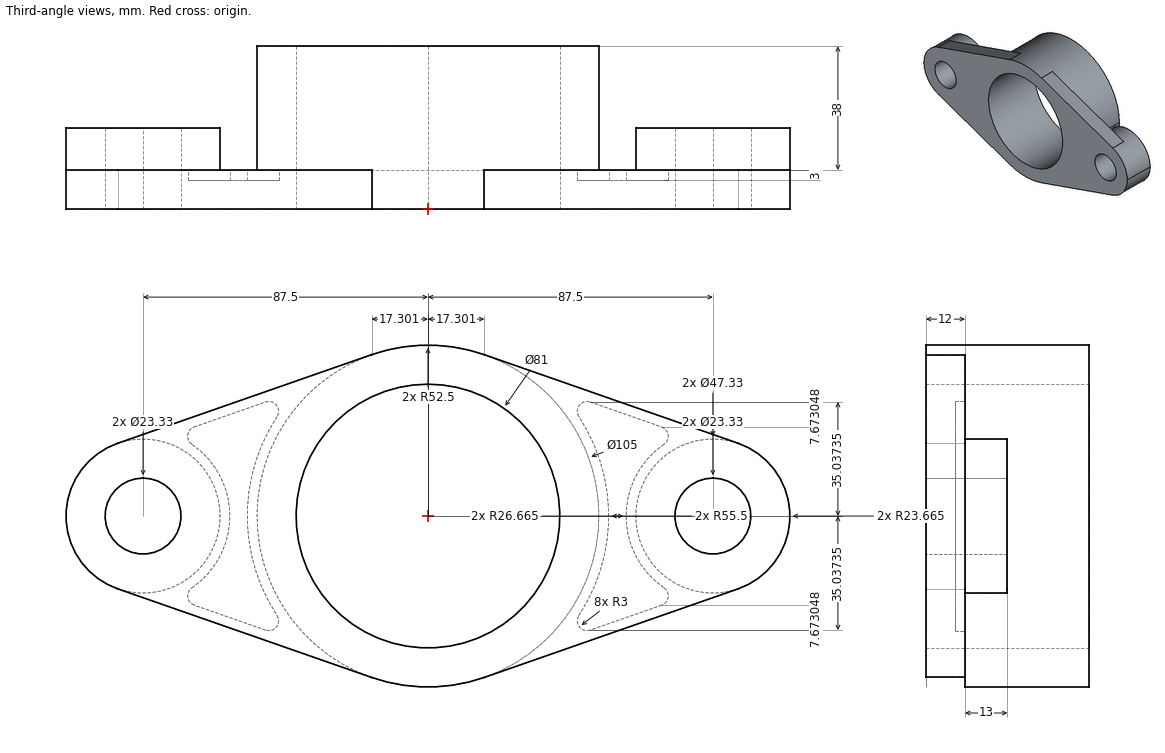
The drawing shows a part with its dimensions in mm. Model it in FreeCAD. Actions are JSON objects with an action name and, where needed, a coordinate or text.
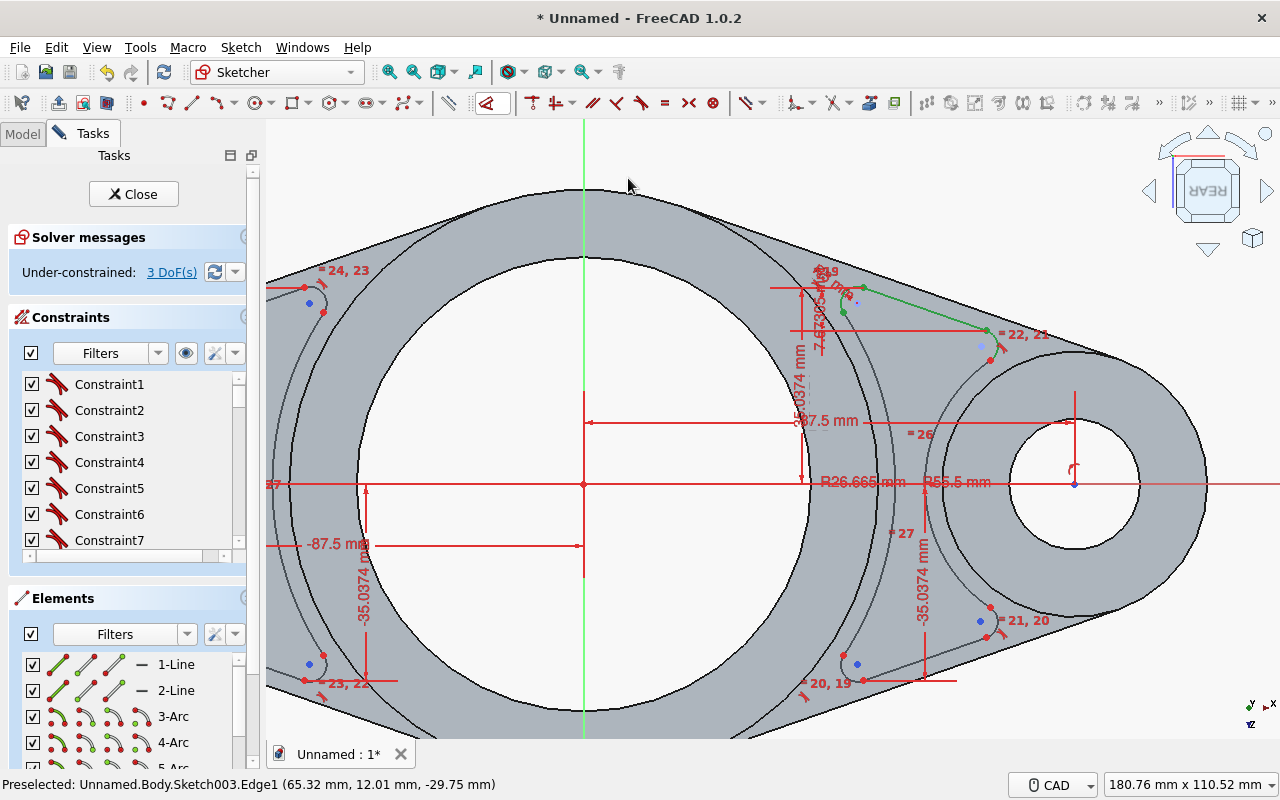
{"action": "left_click", "coordinate": [900, 668]}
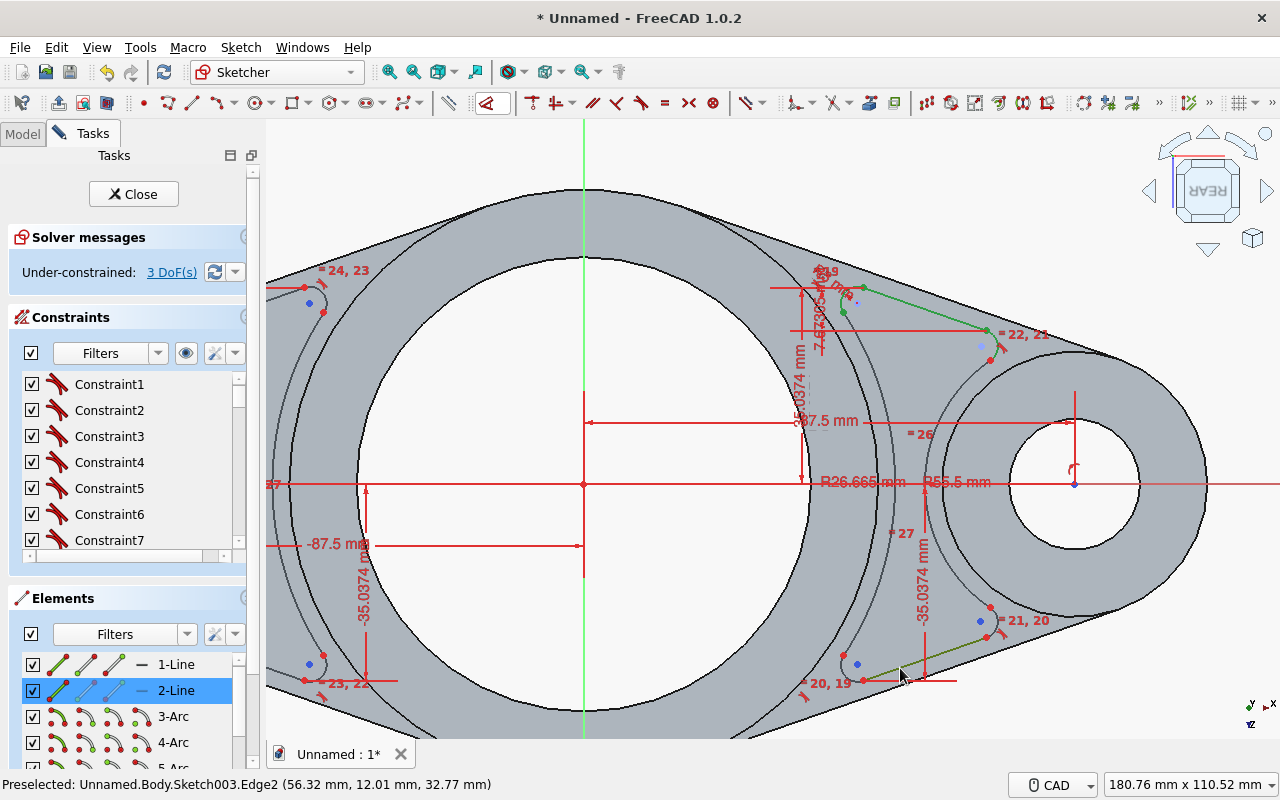
{"action": "key", "text": "i"}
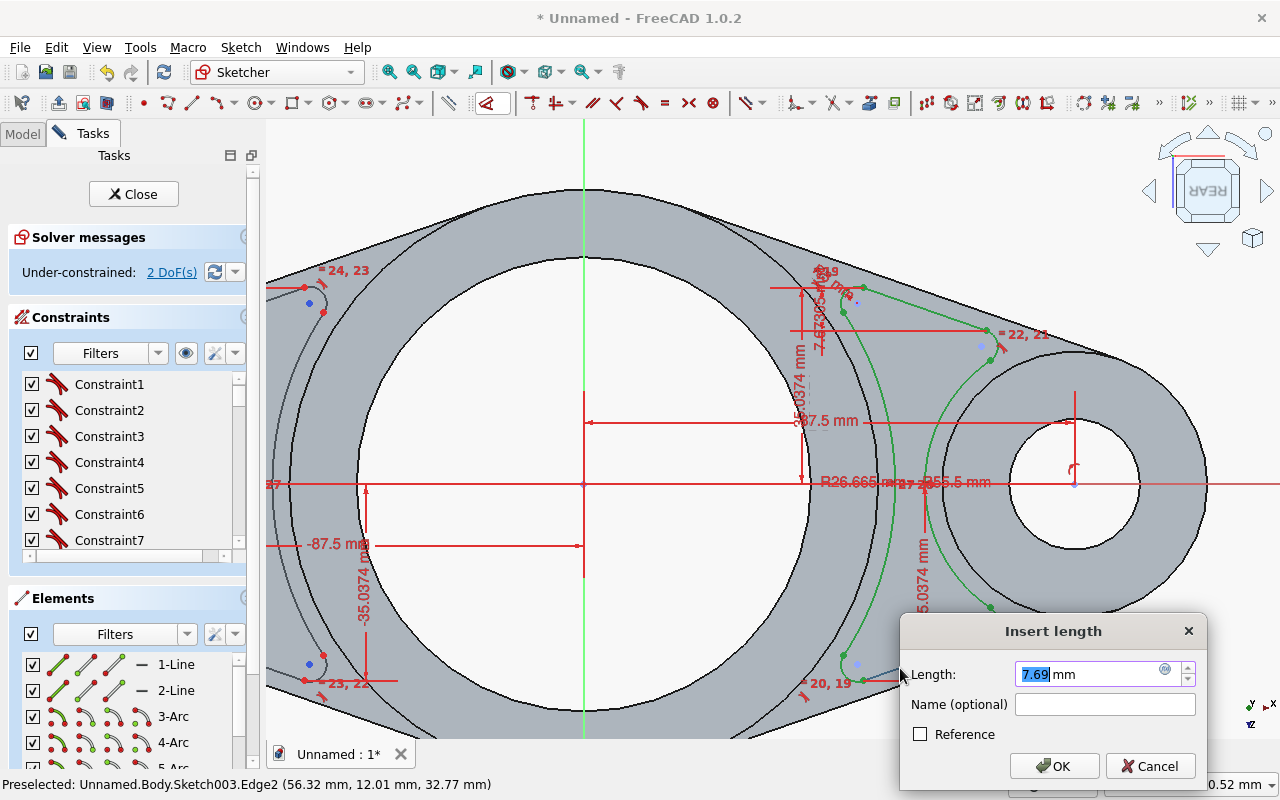
{"action": "type", "text": "7.673048"}
{"action": "key", "text": "Return"}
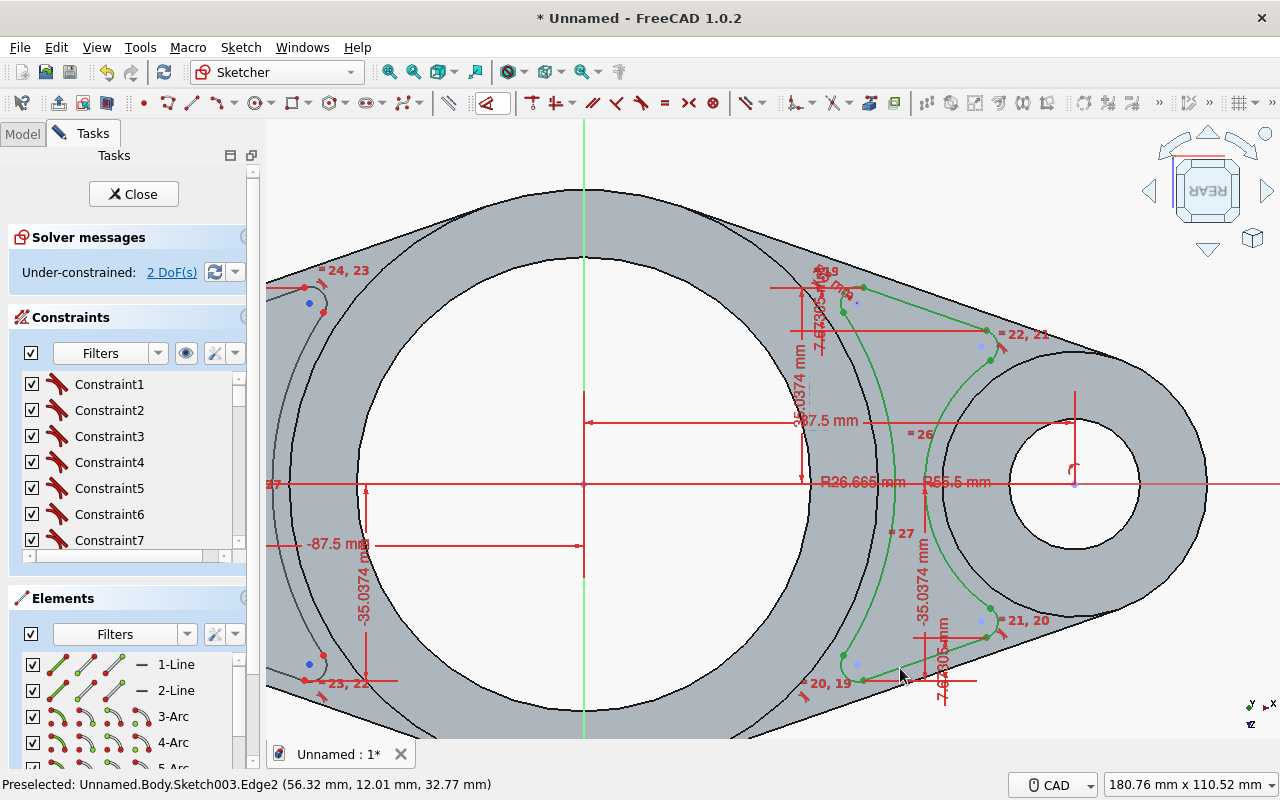
{"action": "scroll", "coordinate": [950, 317], "scroll_direction": "down", "scroll_amount": 2}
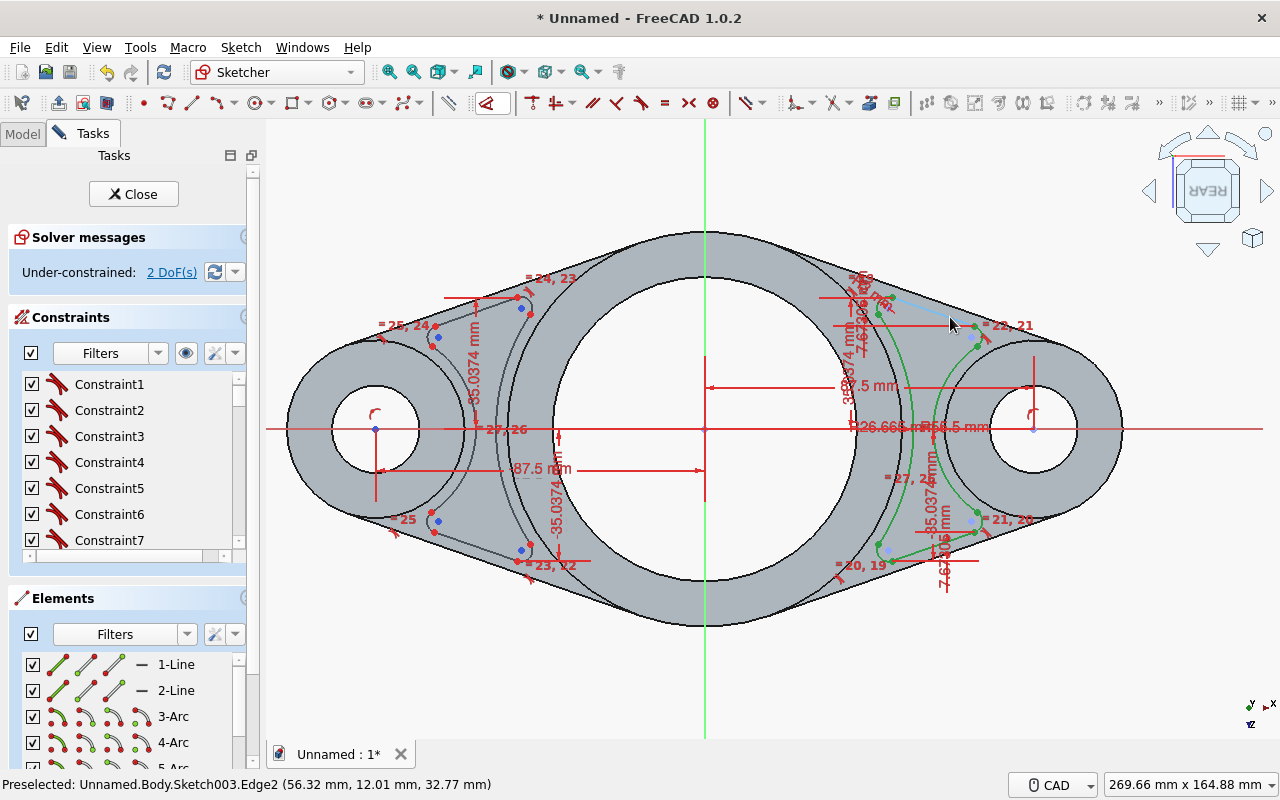
{"action": "scroll", "coordinate": [459, 541], "scroll_direction": "up", "scroll_amount": 2}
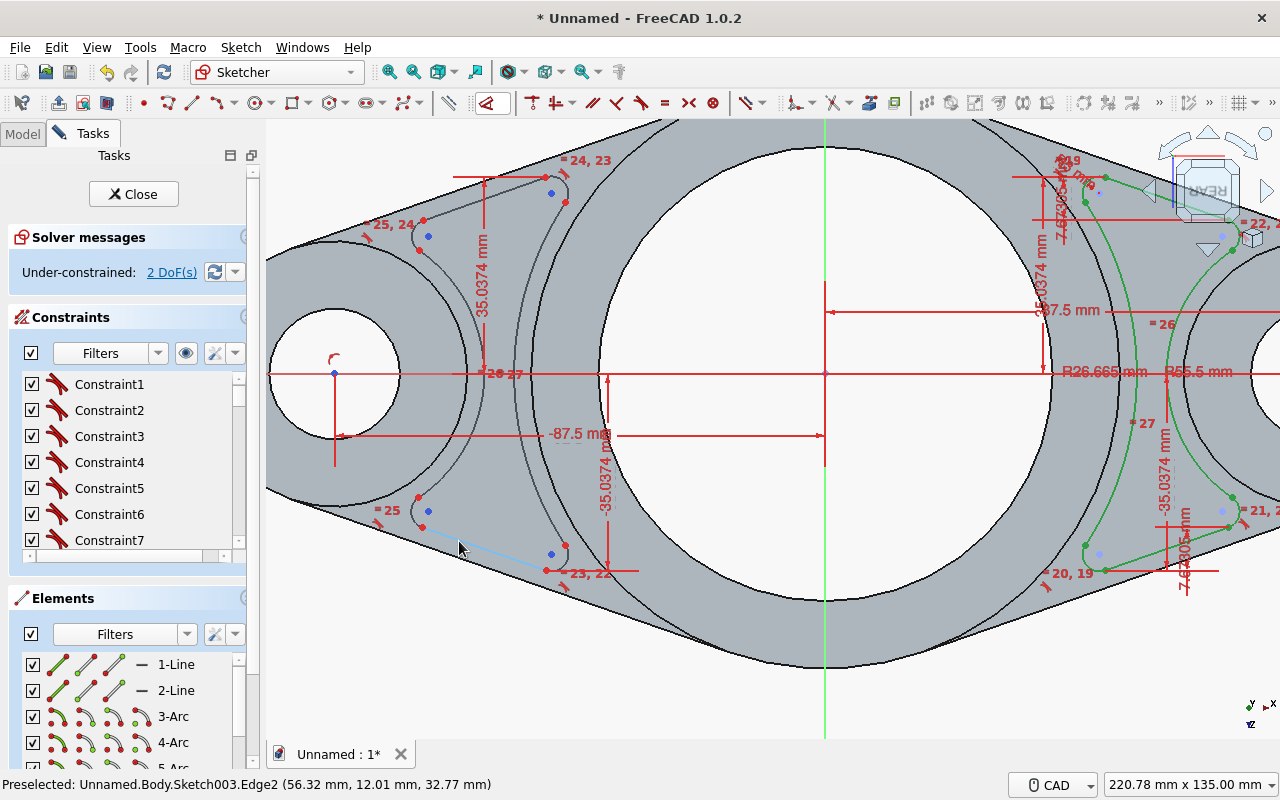
{"action": "left_click", "coordinate": [460, 540]}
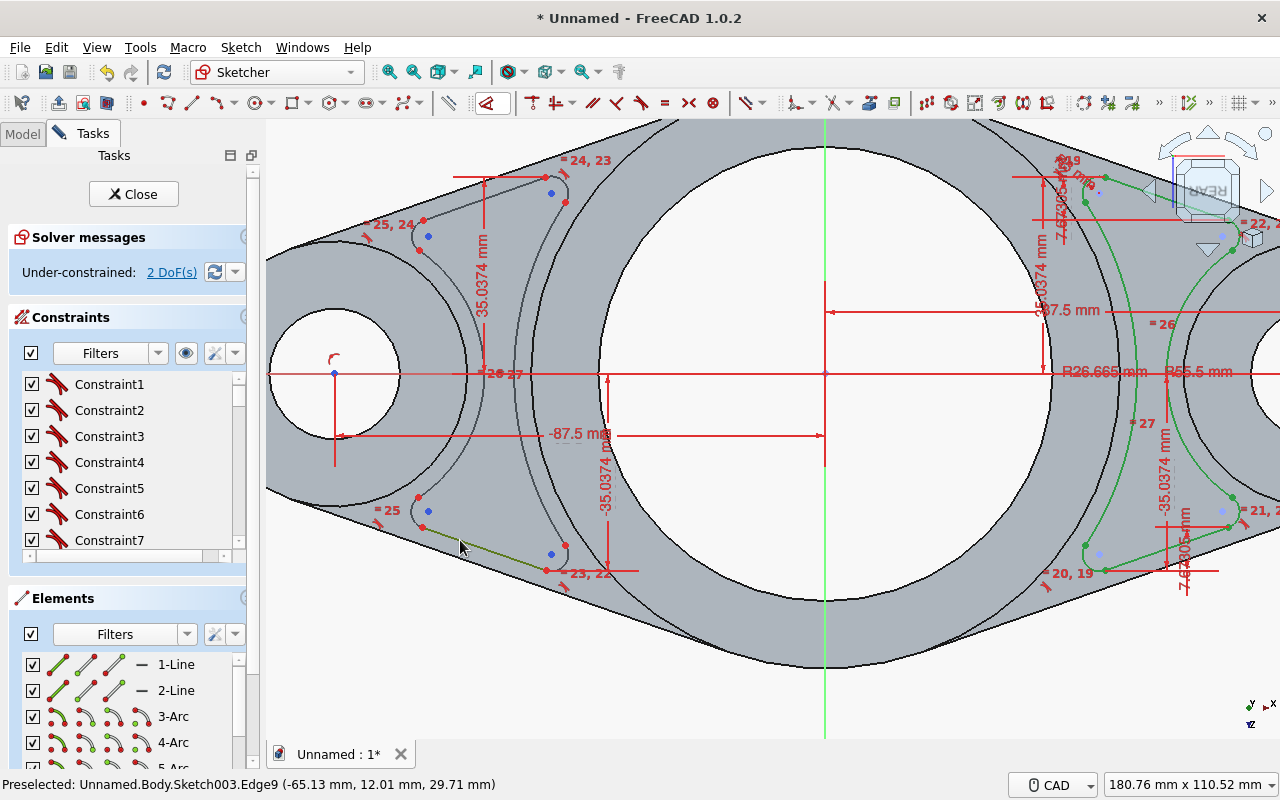
{"action": "left_click", "coordinate": [504, 104]}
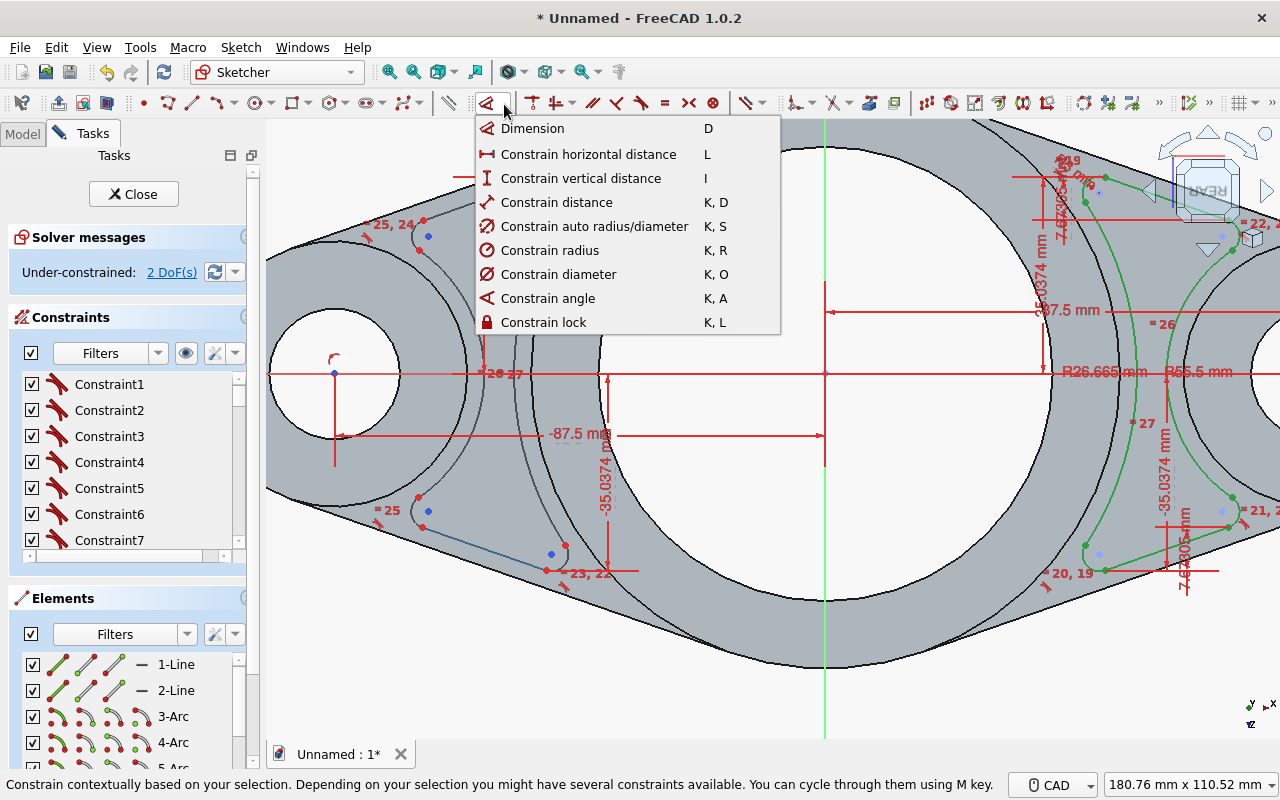
{"action": "left_click", "coordinate": [628, 178]}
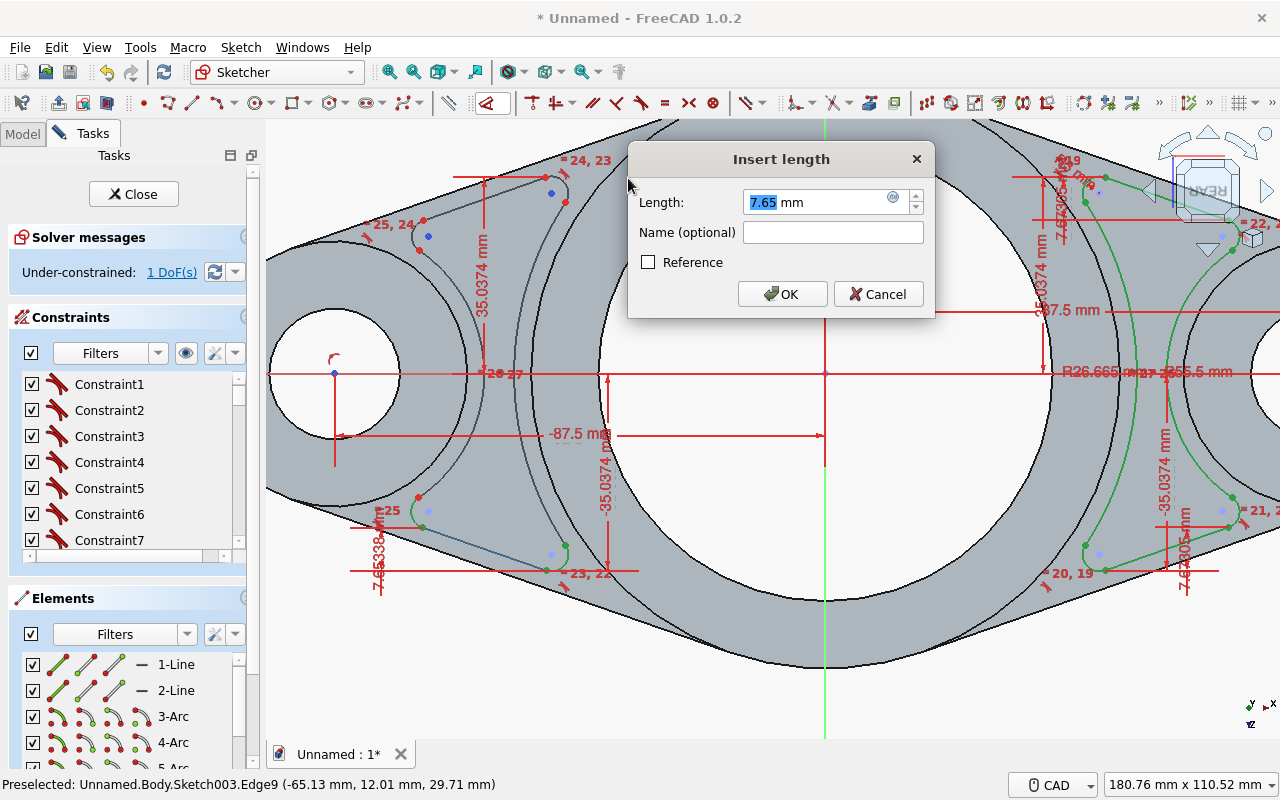
{"action": "type", "text": "7.673048"}
{"action": "key", "text": "Return"}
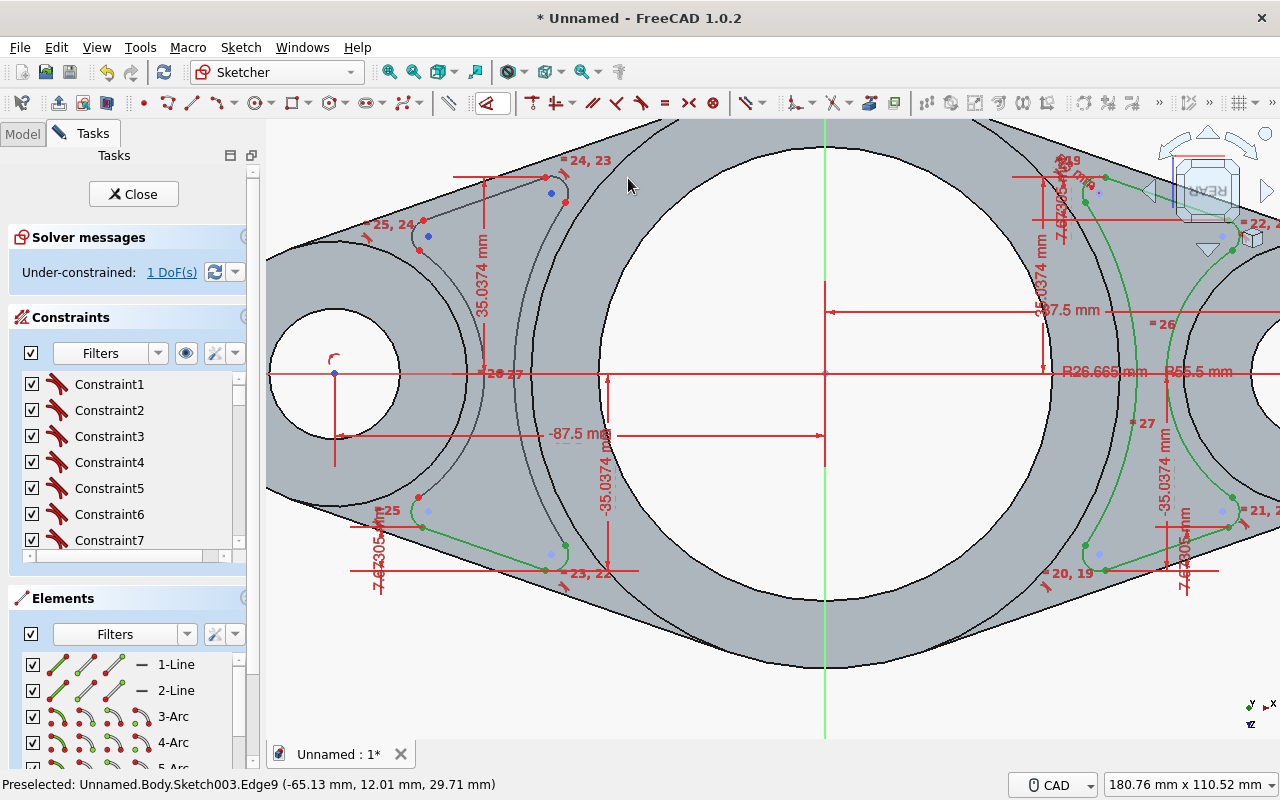
{"action": "left_click", "coordinate": [509, 190]}